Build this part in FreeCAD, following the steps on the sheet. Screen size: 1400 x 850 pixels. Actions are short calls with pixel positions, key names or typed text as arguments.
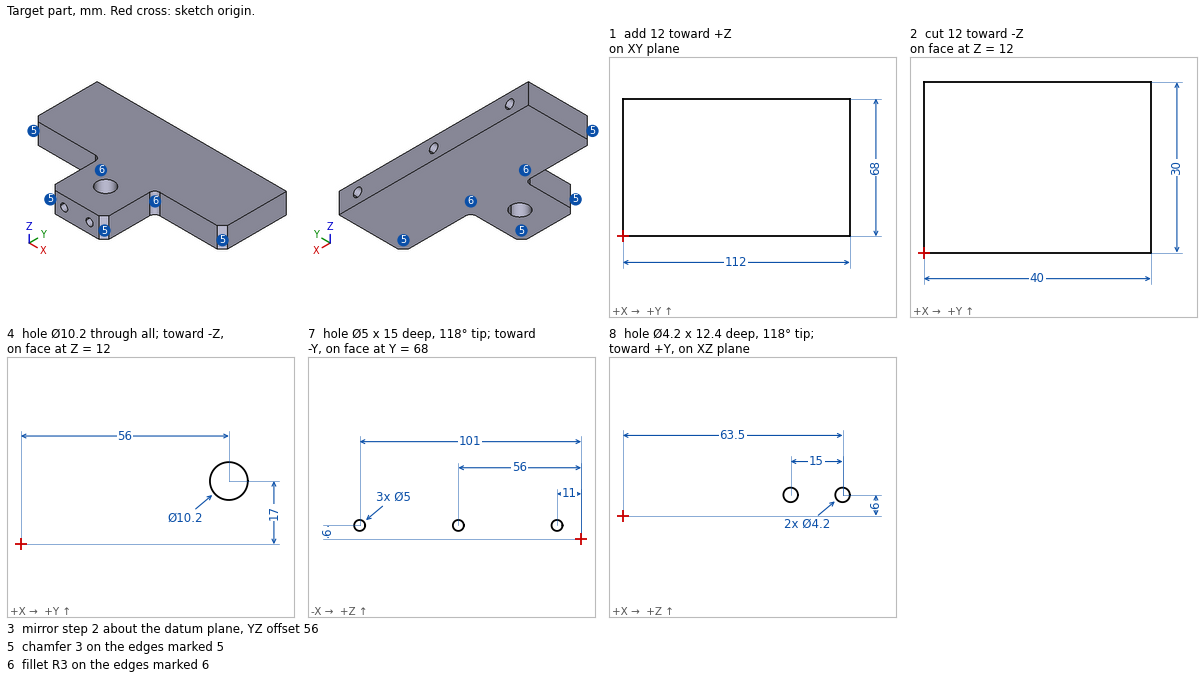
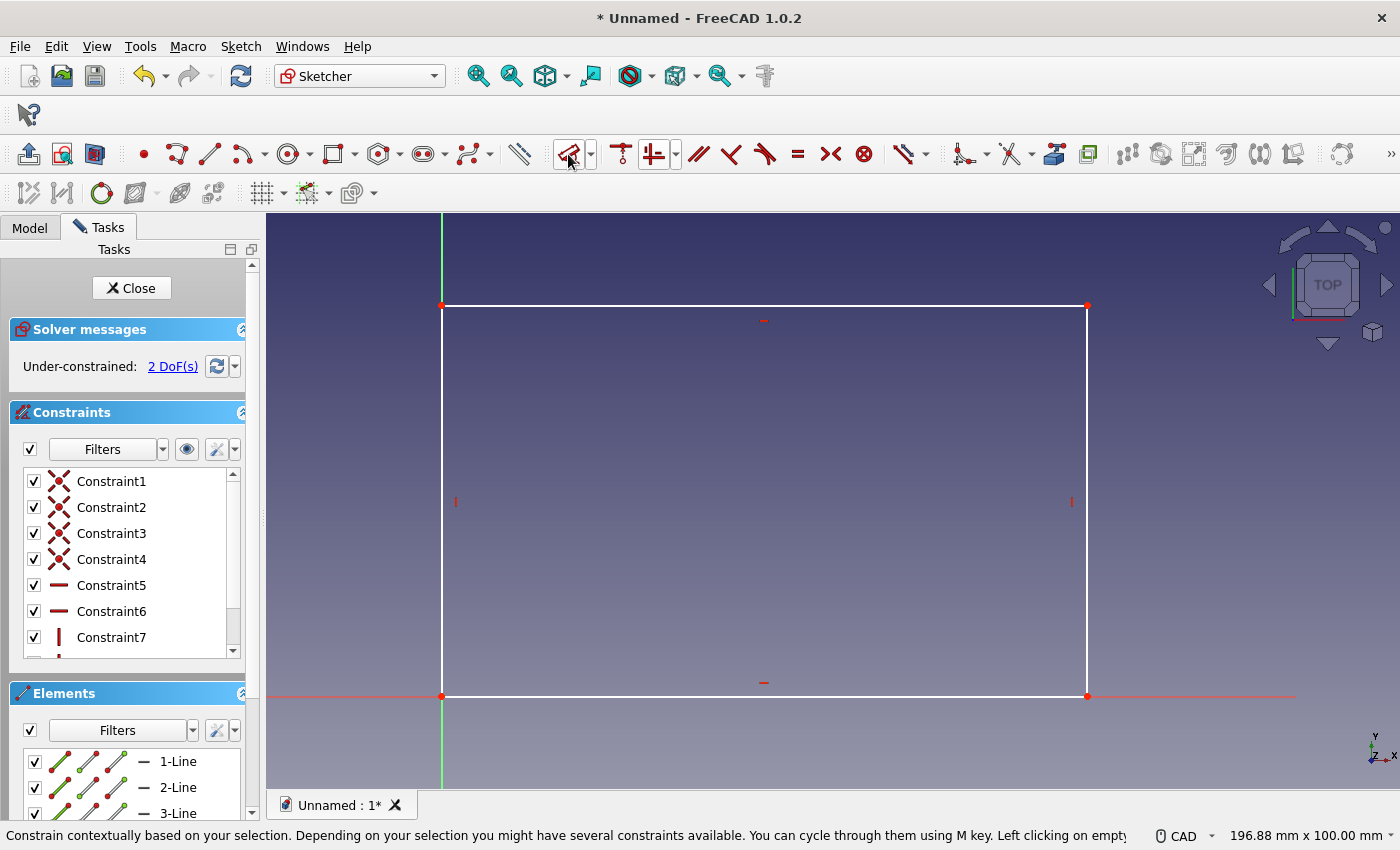
click(1087, 579)
click(1121, 501)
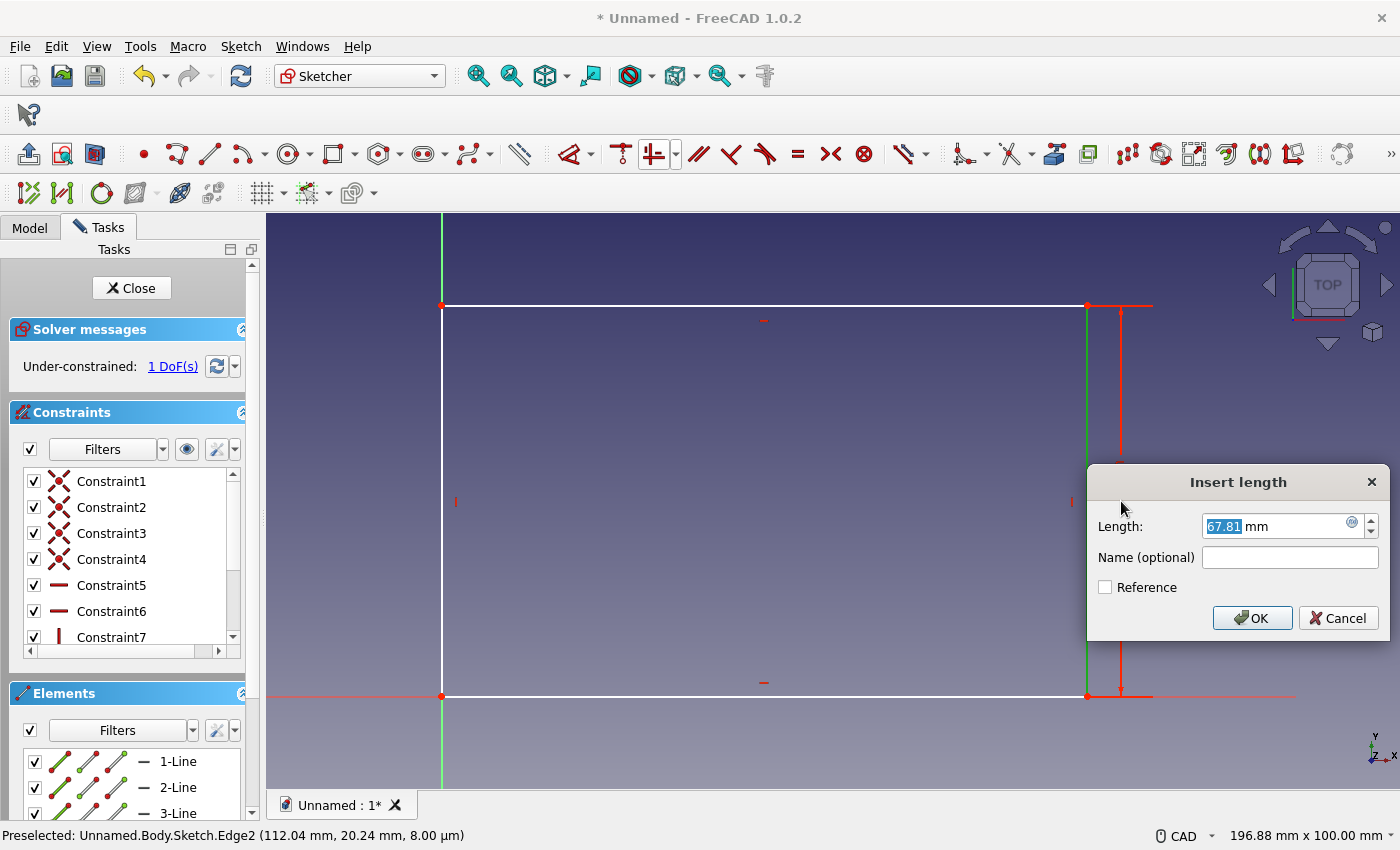
text(68)
key(Return)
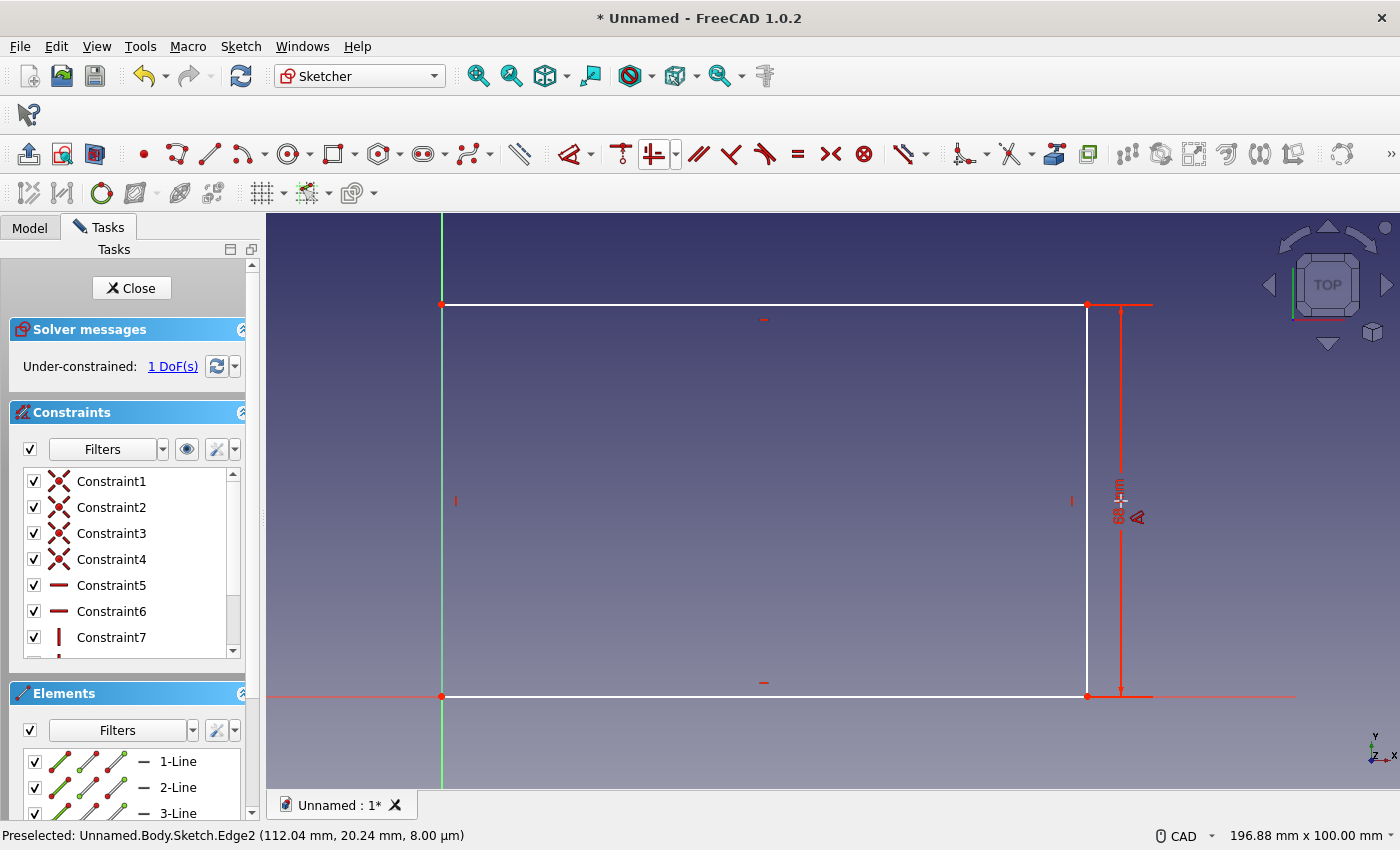
click(635, 697)
click(764, 731)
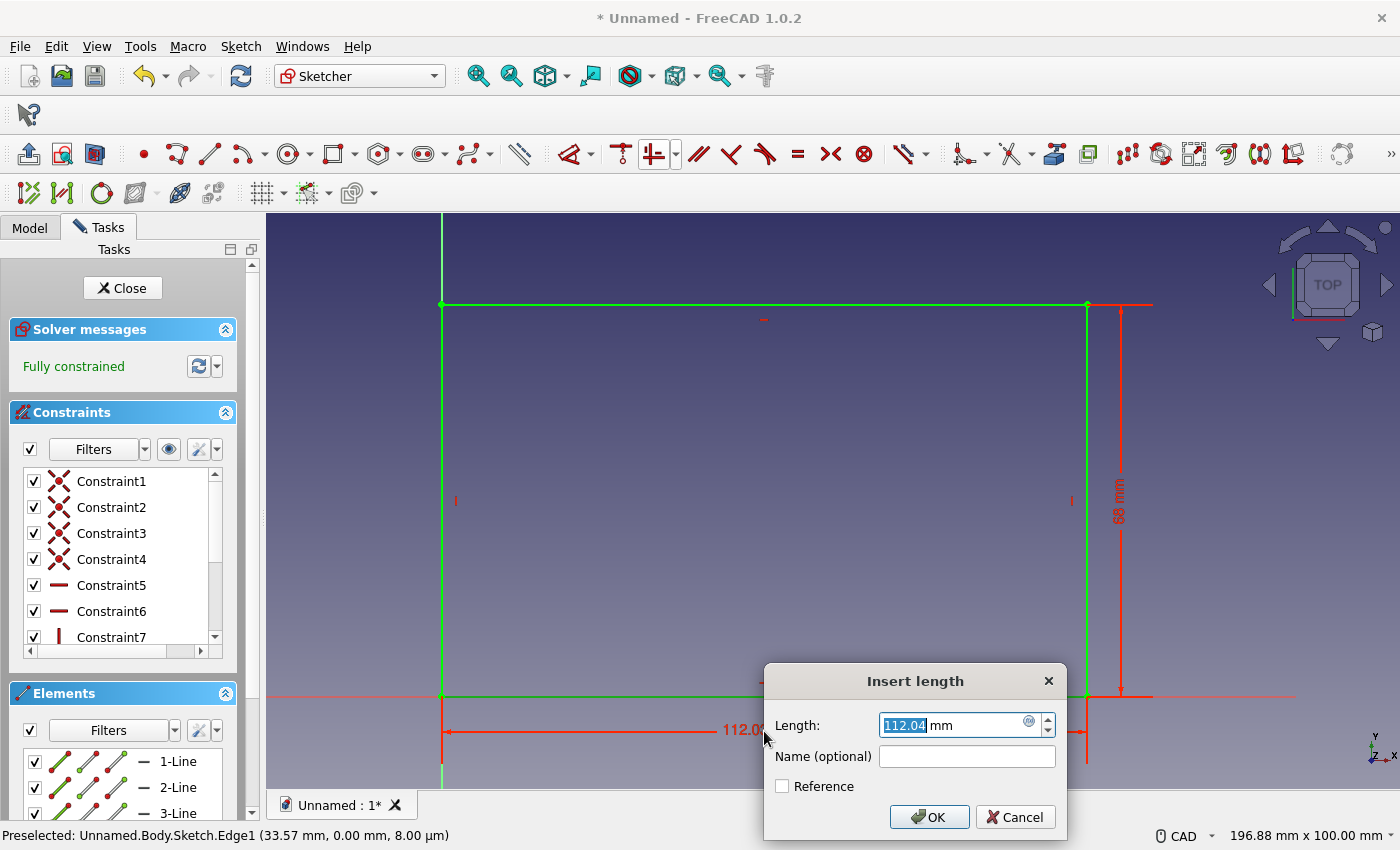
text(112)
key(Return)
key(Escape)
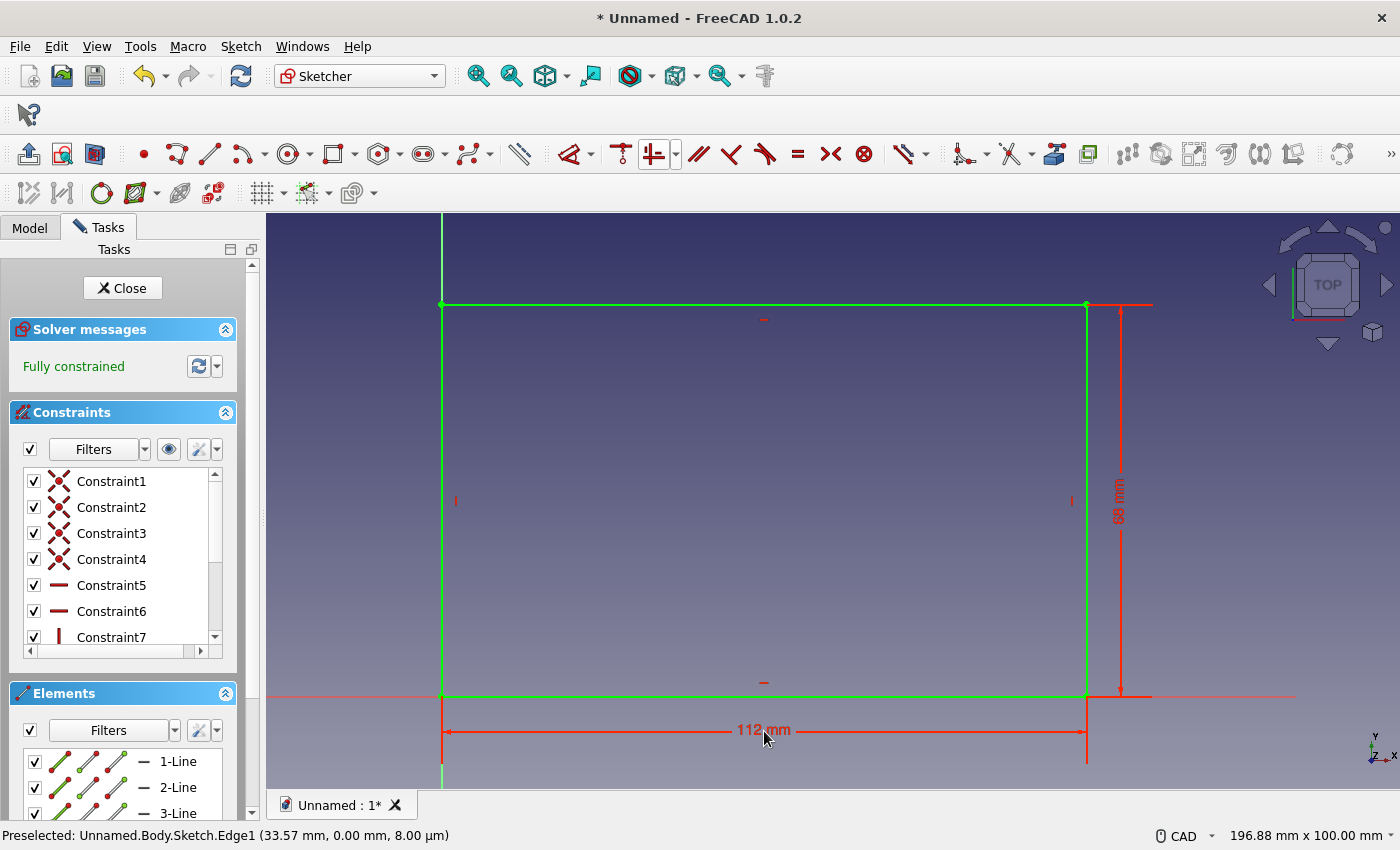
click(123, 288)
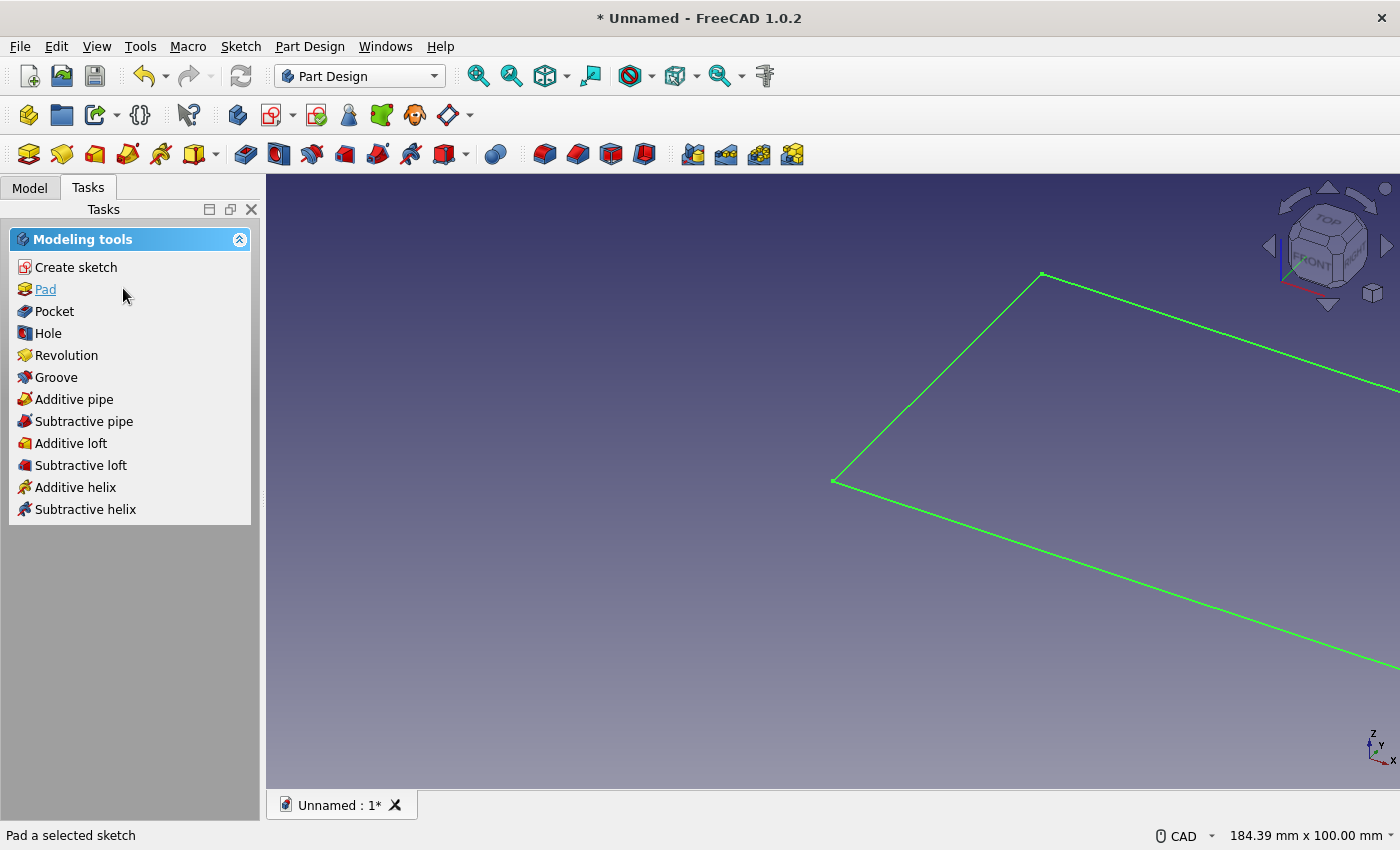
click(29, 154)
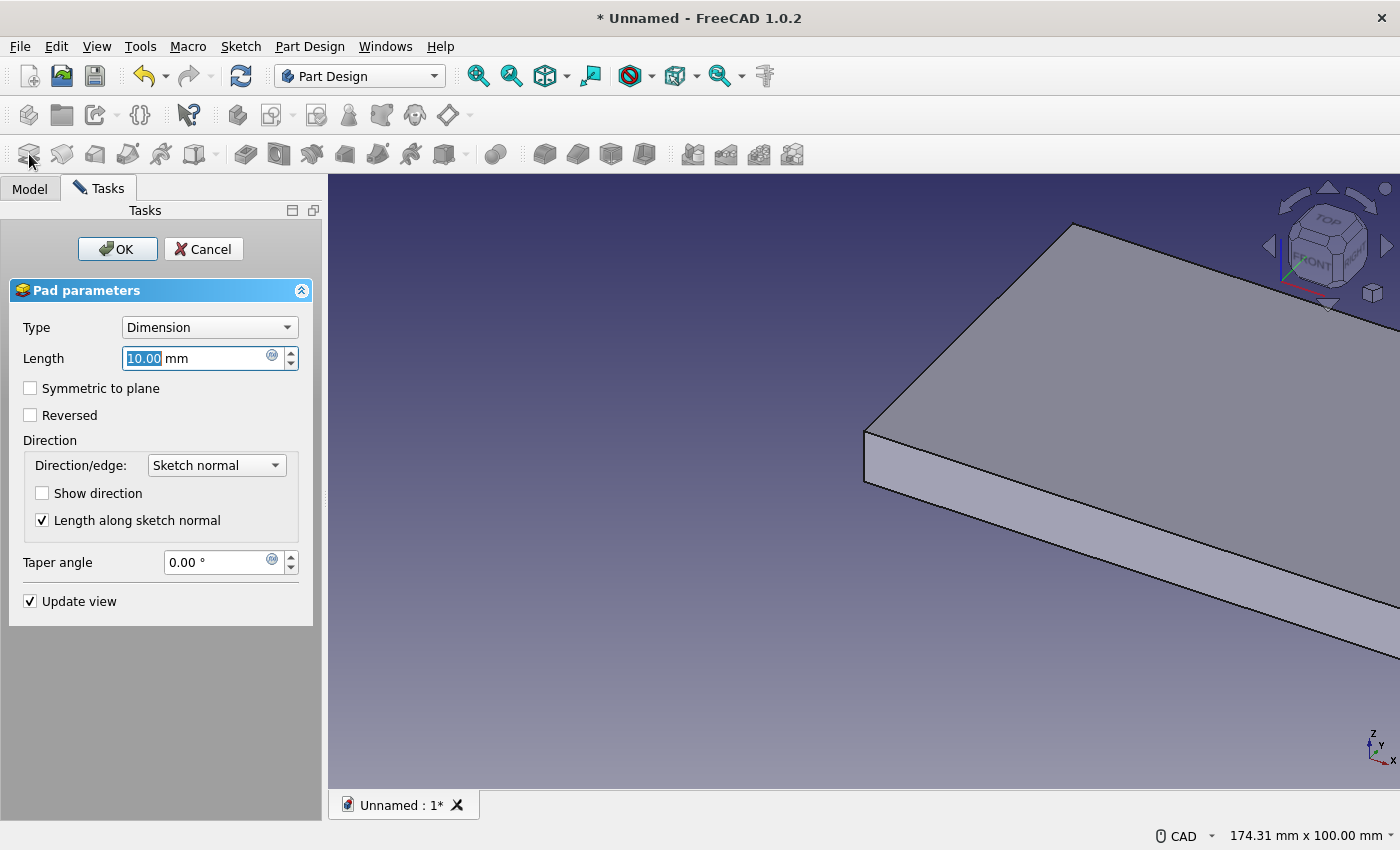
text(12)
key(Tab)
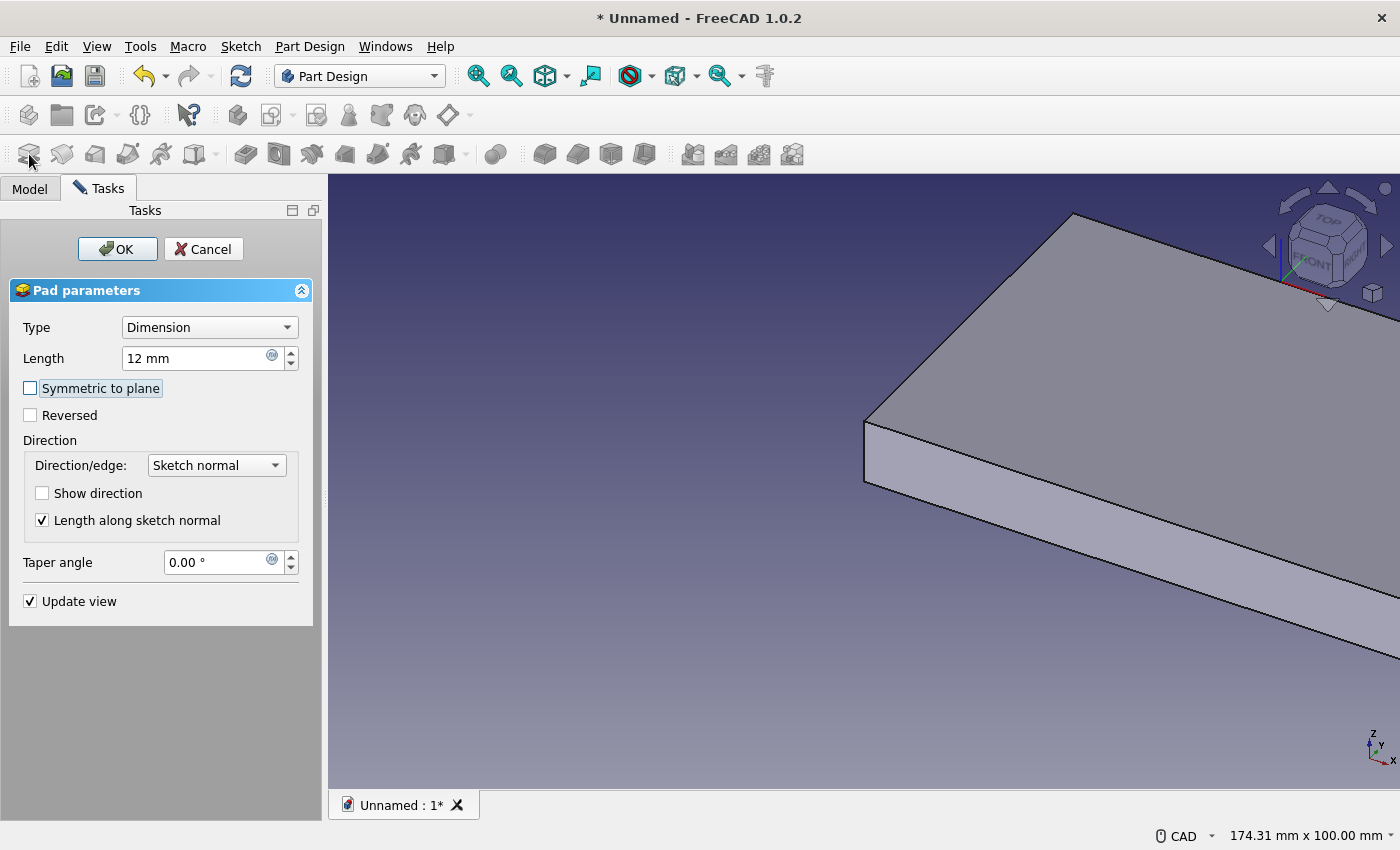
click(118, 249)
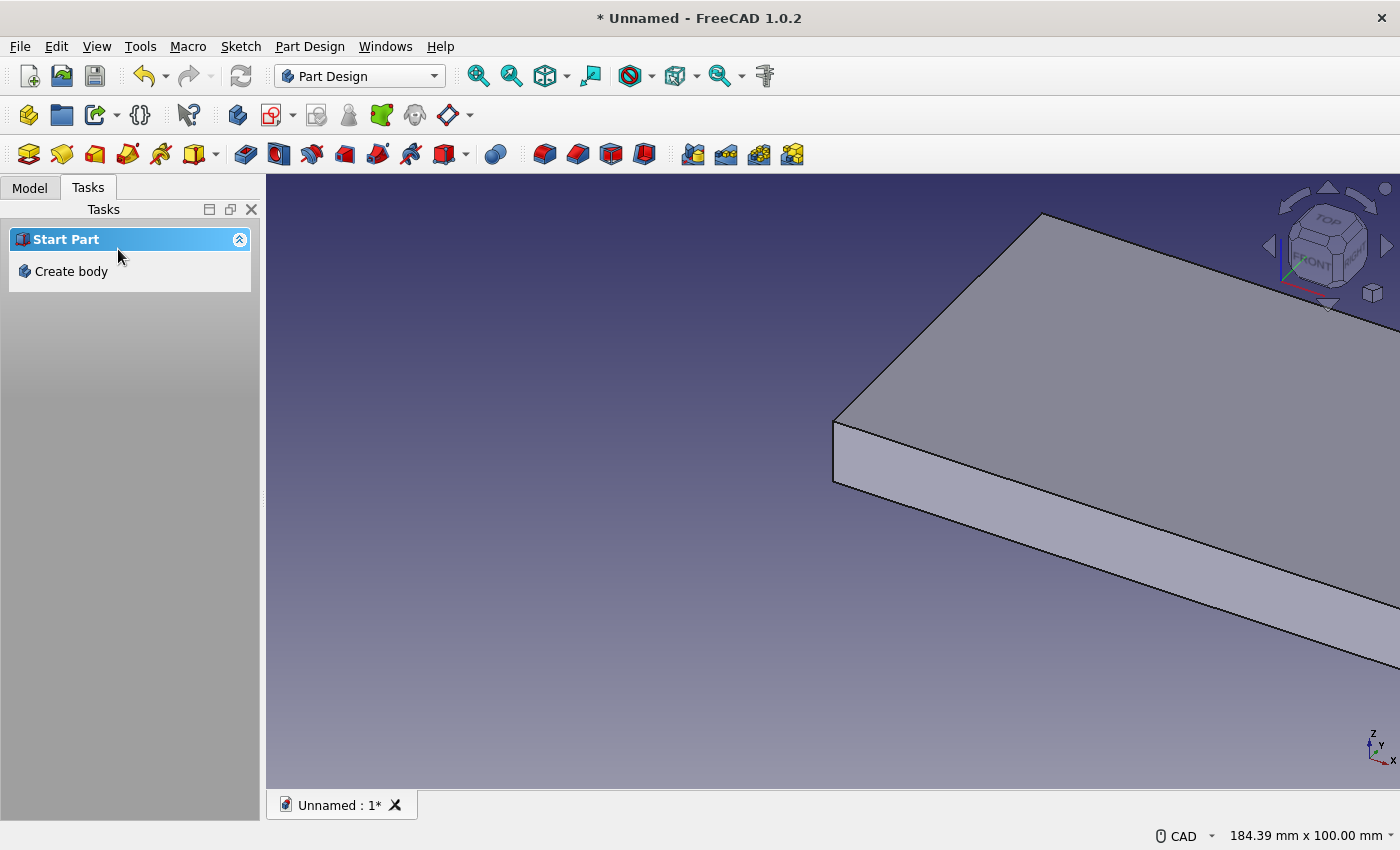
click(479, 76)